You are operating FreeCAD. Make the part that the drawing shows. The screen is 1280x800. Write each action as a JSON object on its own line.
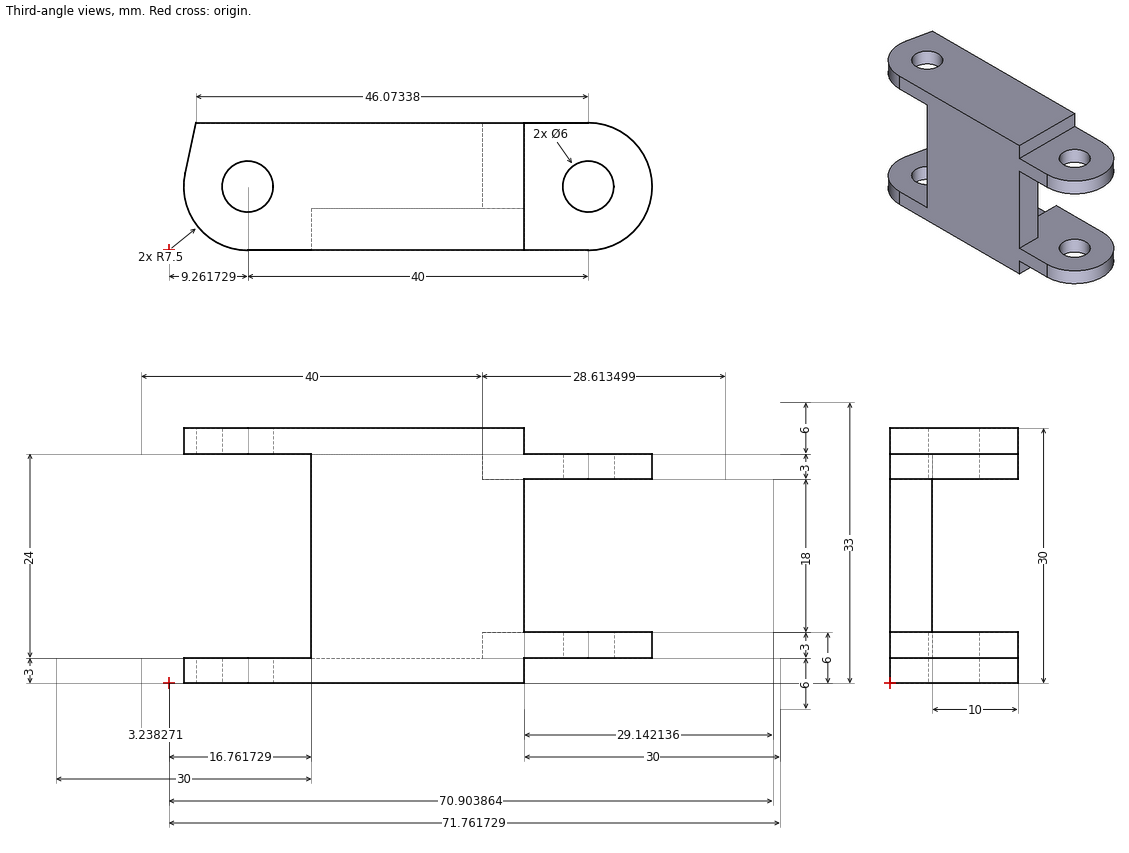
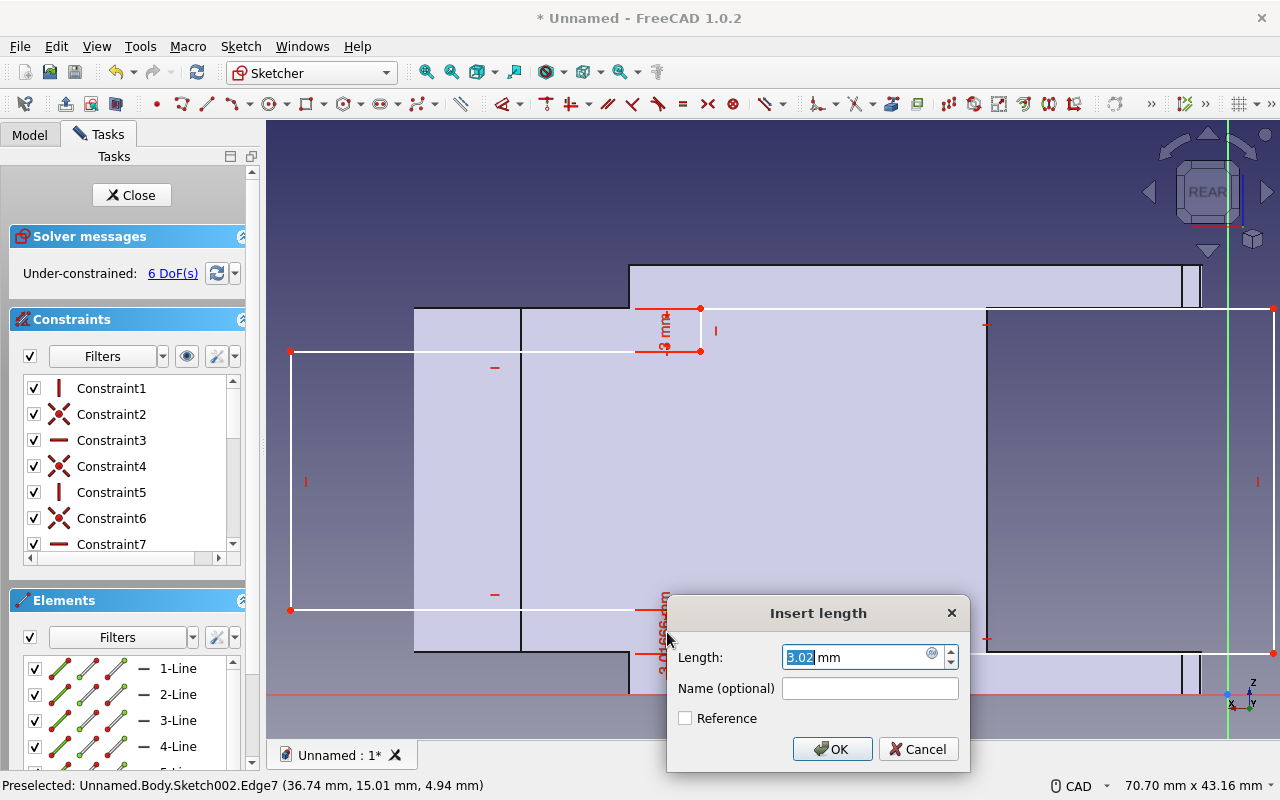
{"action": "type", "text": "3"}
{"action": "key", "text": "Return"}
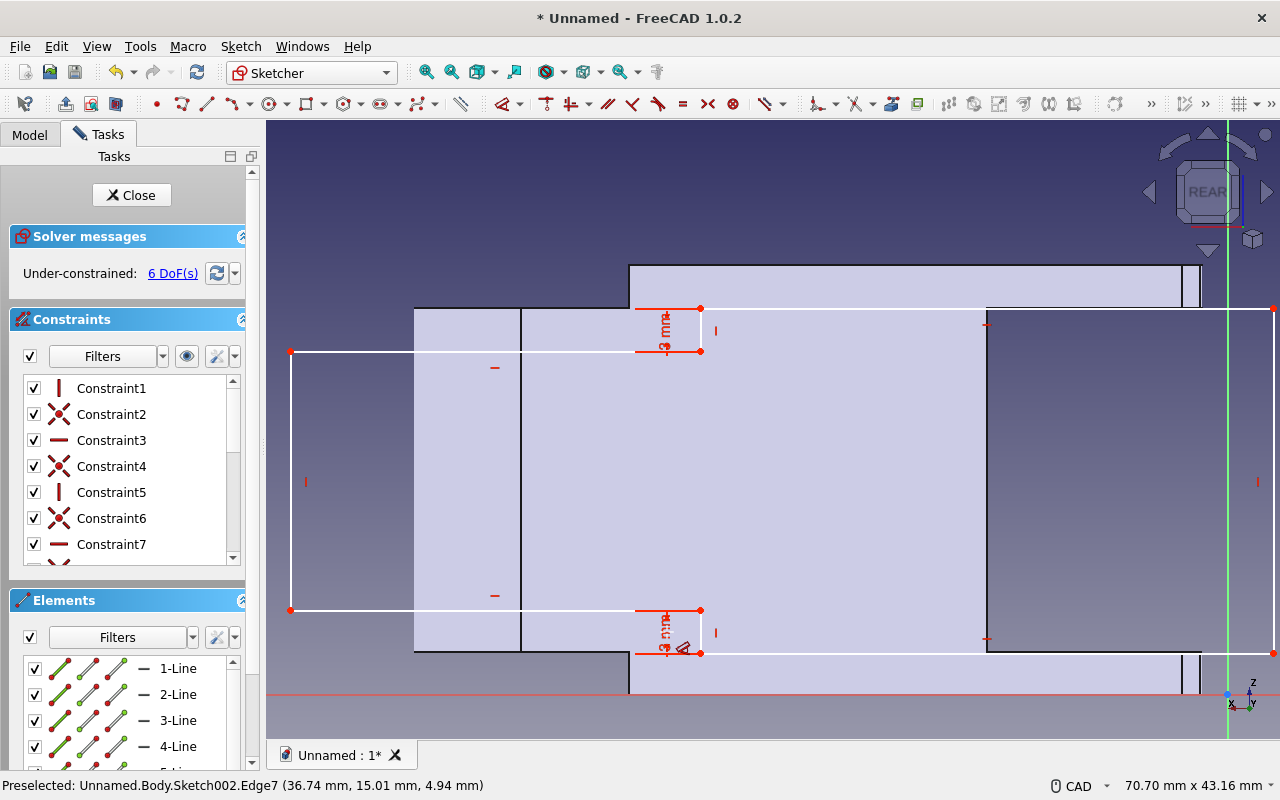
{"action": "scroll", "coordinate": [610, 342], "scroll_direction": "down", "scroll_amount": 3}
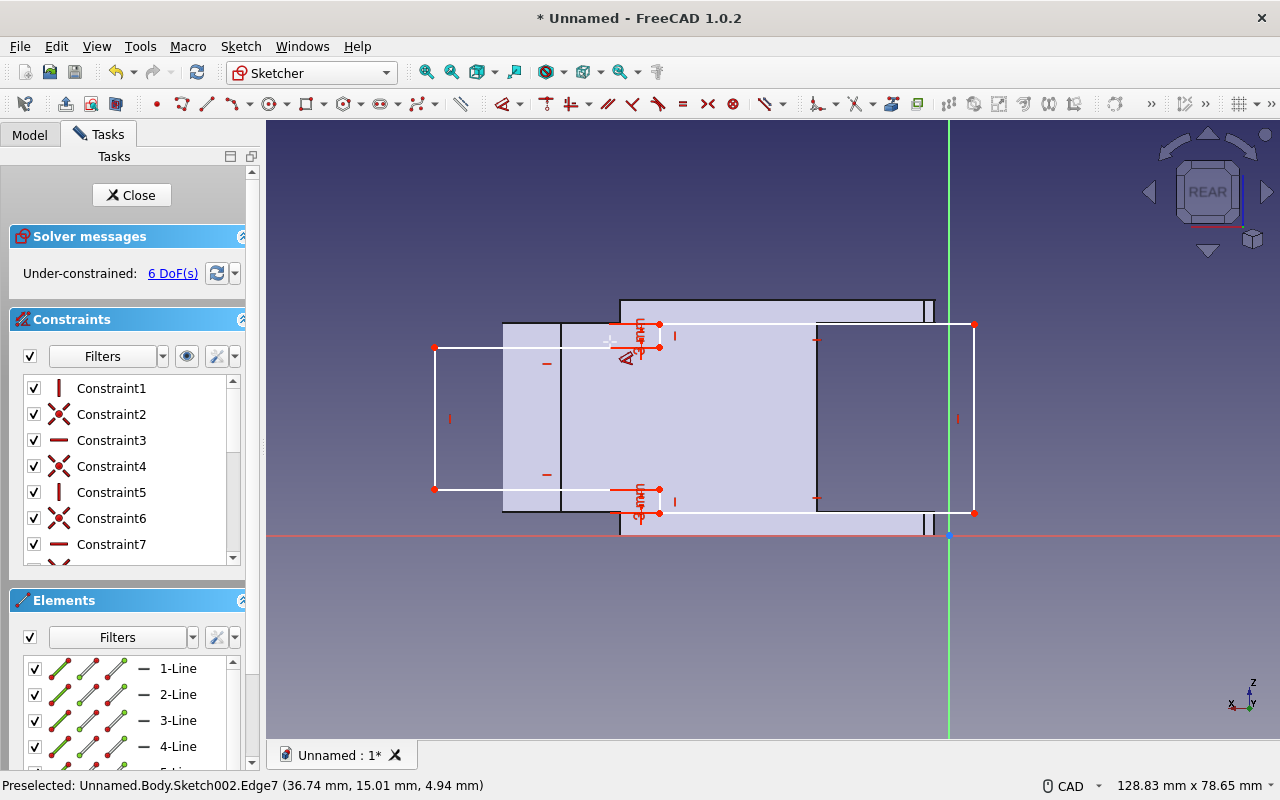
{"action": "left_click", "coordinate": [974, 456]}
{"action": "left_click", "coordinate": [1008, 419]}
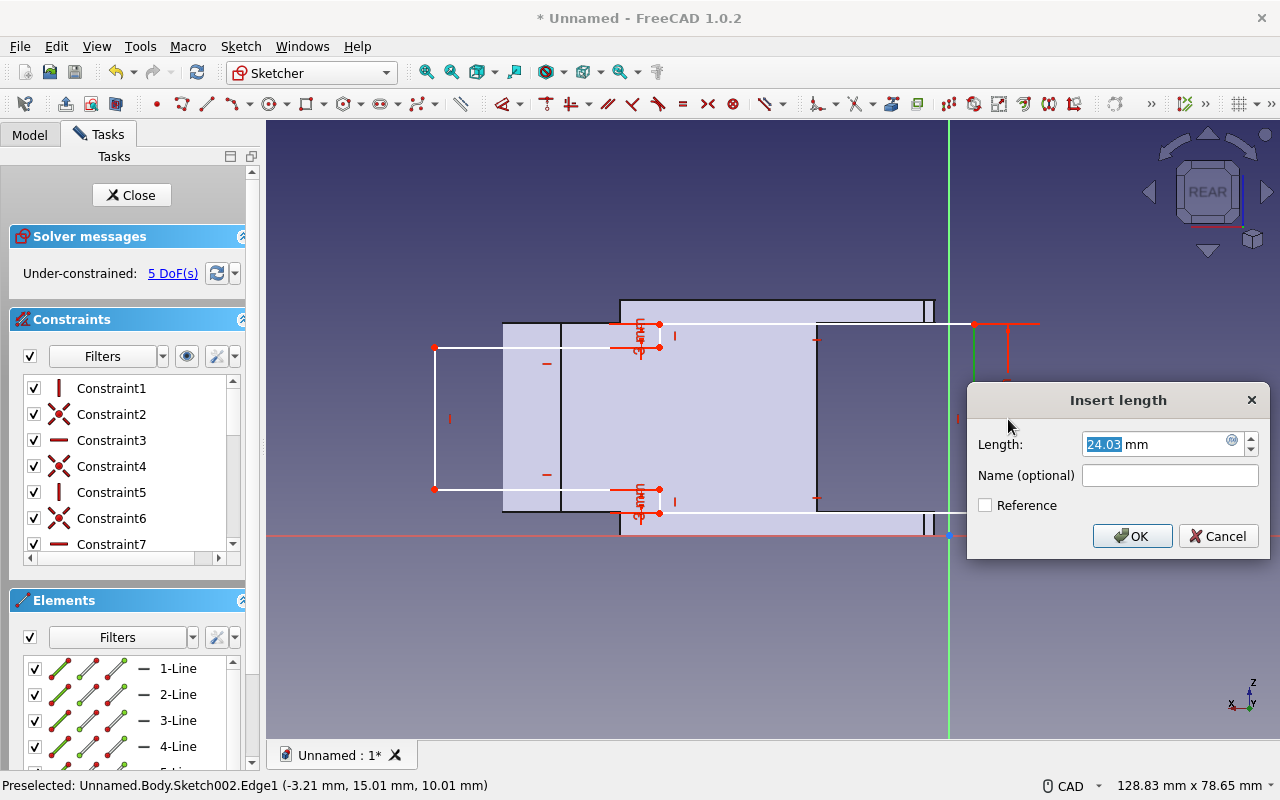
{"action": "type", "text": "24"}
{"action": "key", "text": "Return"}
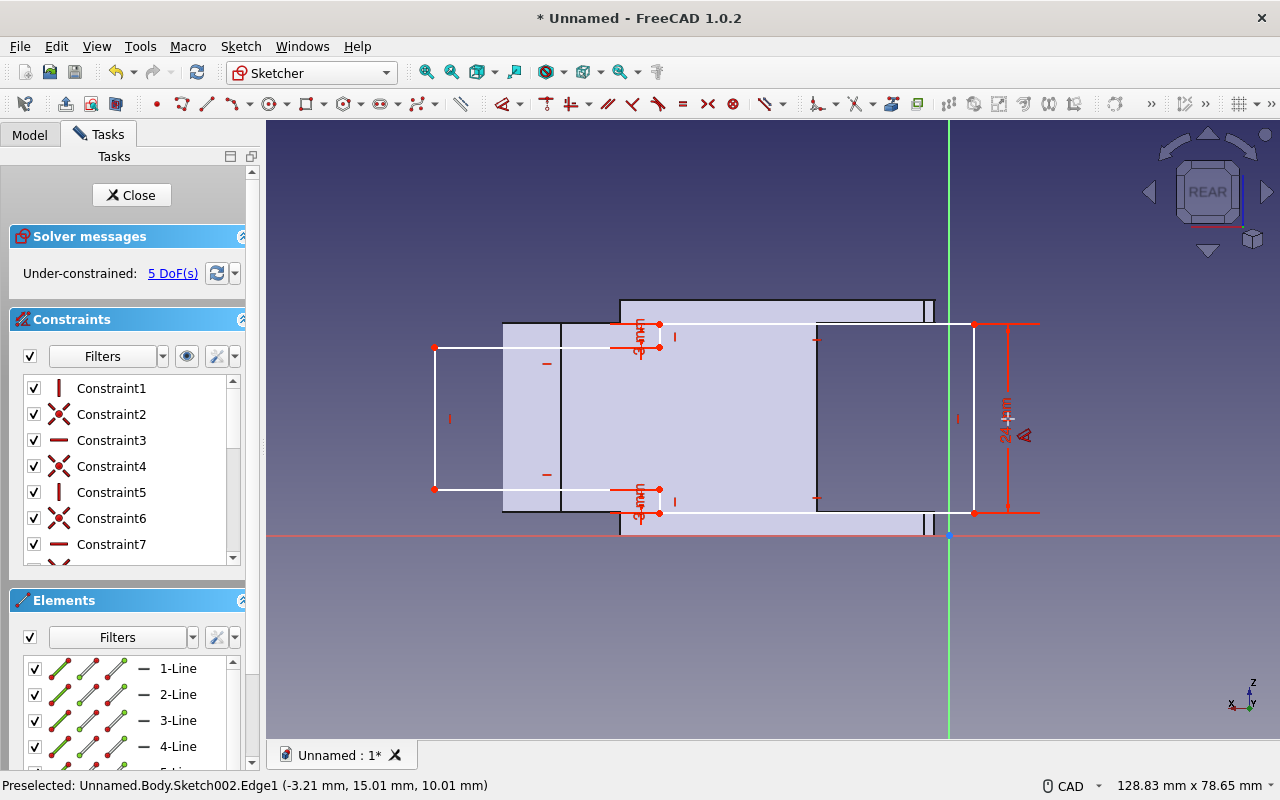
{"action": "left_click", "coordinate": [880, 324]}
{"action": "left_click", "coordinate": [817, 290]}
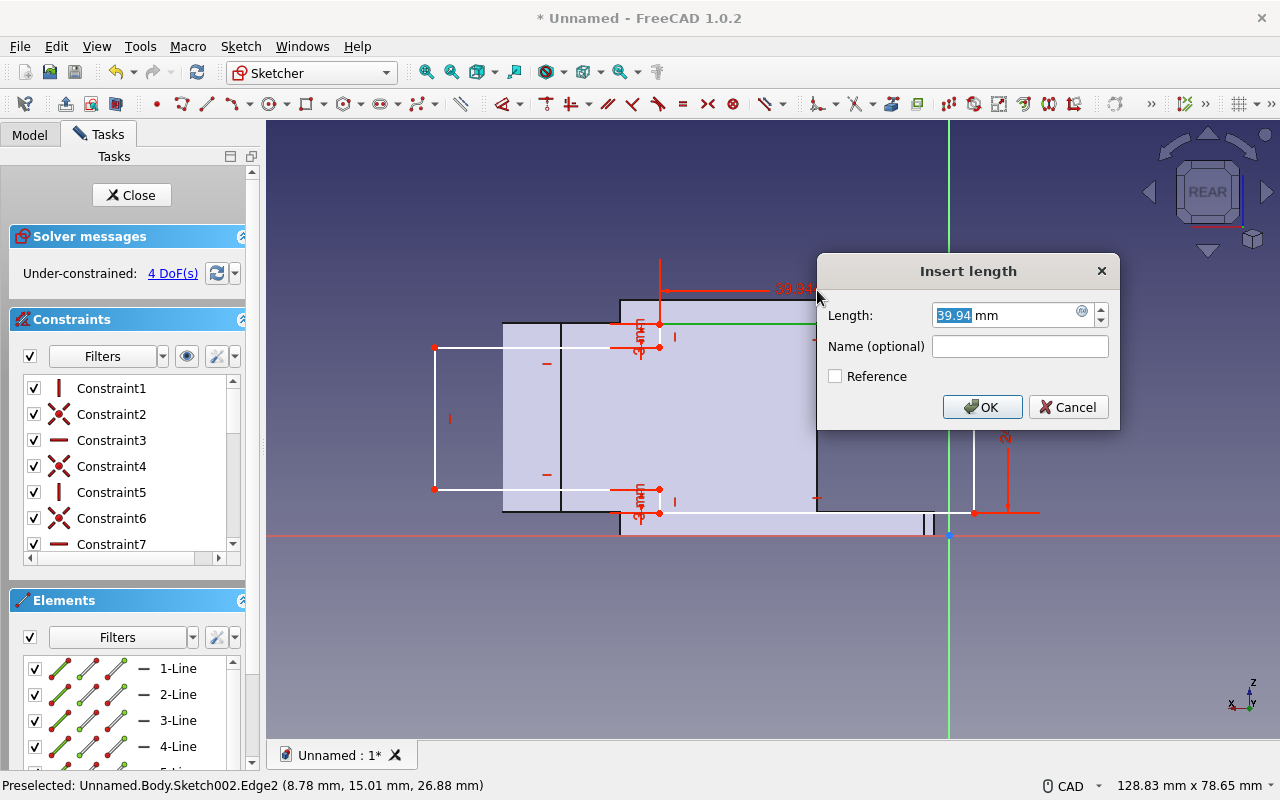
{"action": "type", "text": "40"}
{"action": "key", "text": "Return"}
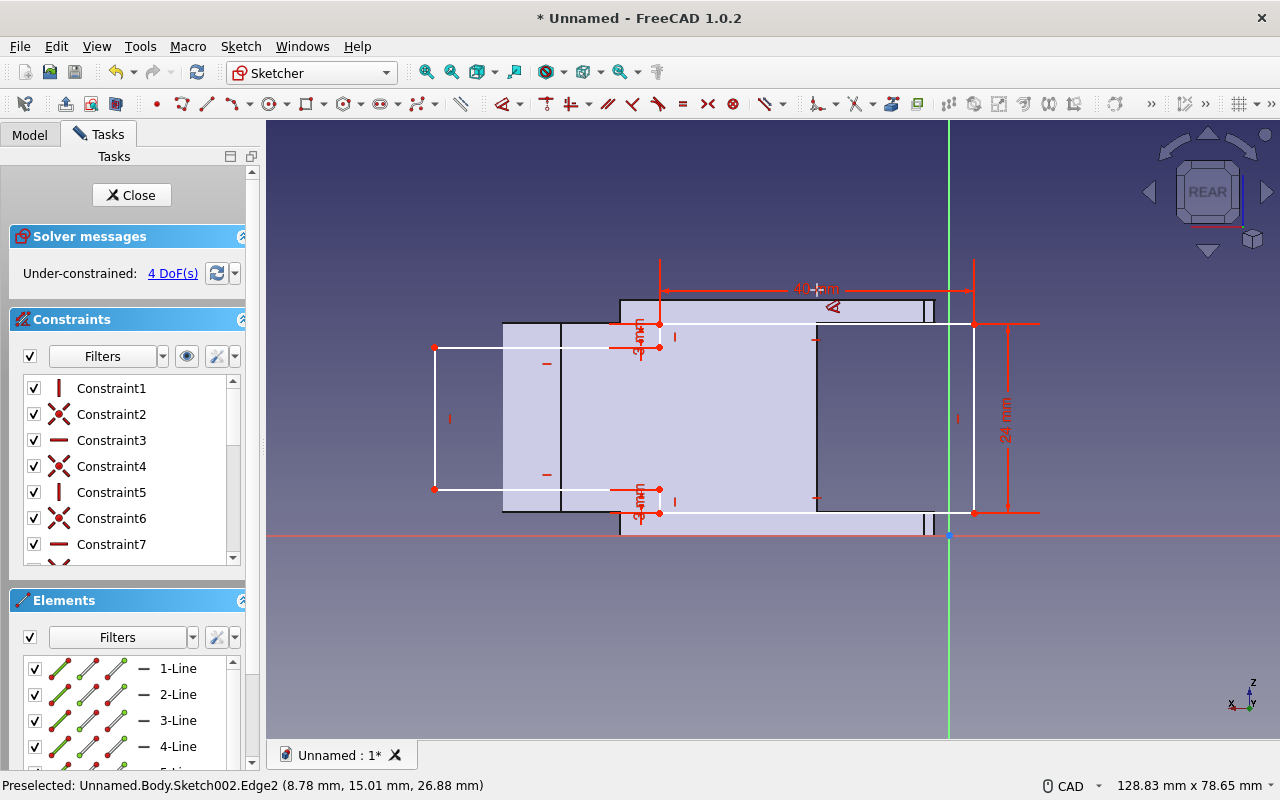
{"action": "left_click", "coordinate": [754, 513]}
{"action": "left_click", "coordinate": [817, 479]}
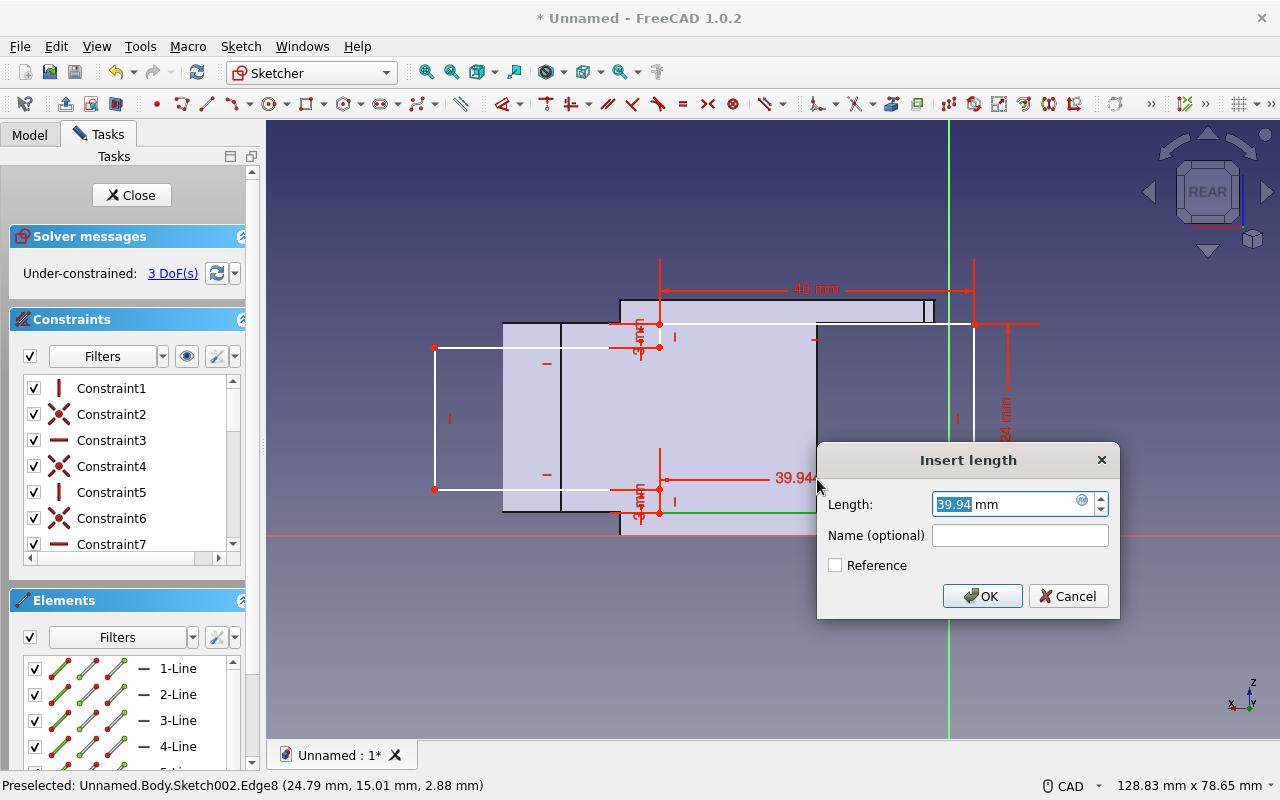
{"action": "type", "text": "40"}
{"action": "key", "text": "Return"}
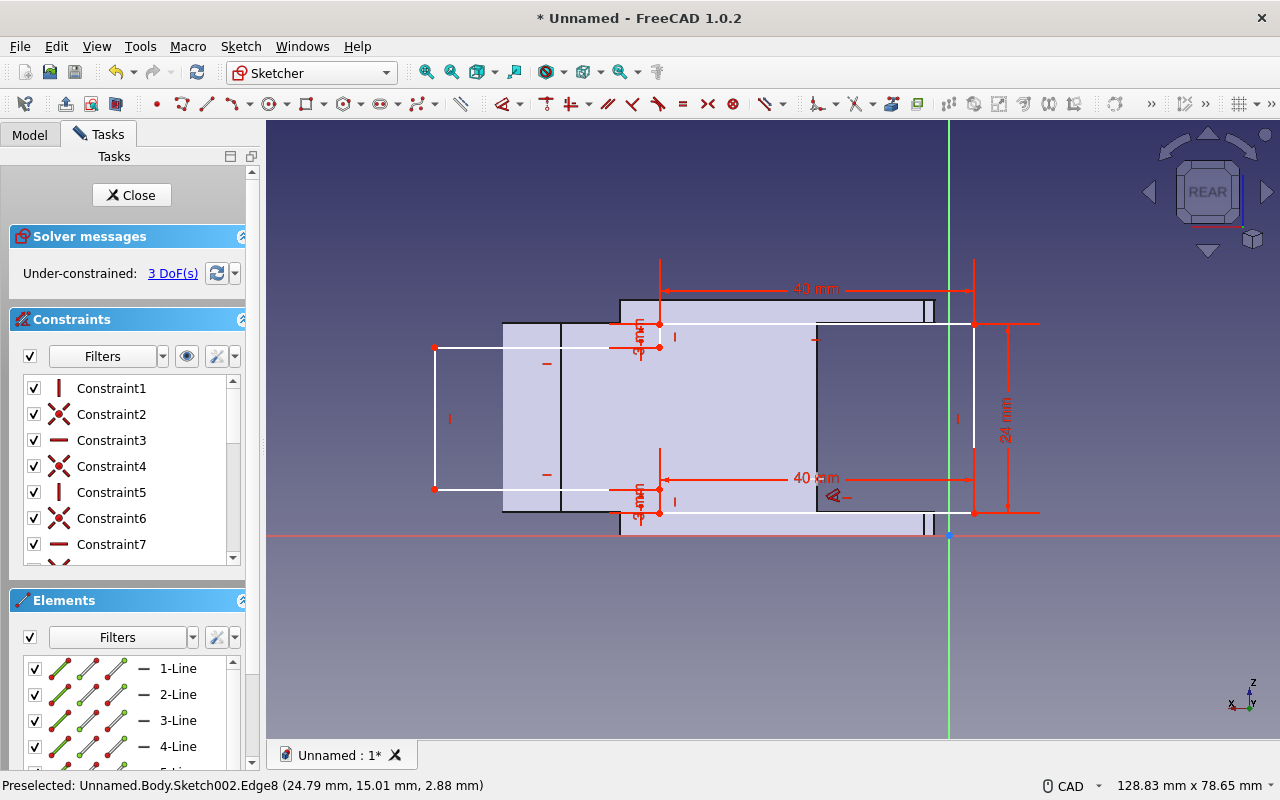
{"action": "scroll", "coordinate": [974, 513], "scroll_direction": "up", "scroll_amount": 3}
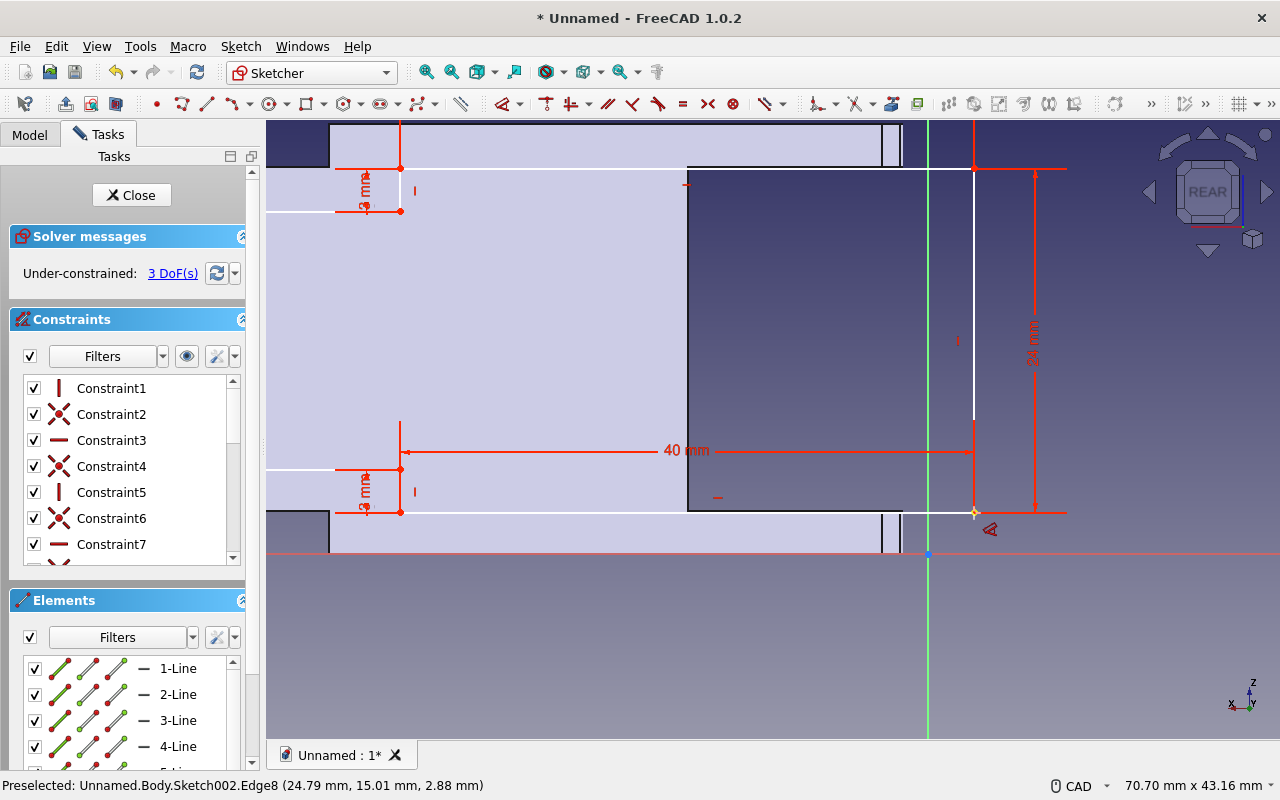
{"action": "left_click", "coordinate": [974, 513]}
{"action": "left_click", "coordinate": [1008, 533]}